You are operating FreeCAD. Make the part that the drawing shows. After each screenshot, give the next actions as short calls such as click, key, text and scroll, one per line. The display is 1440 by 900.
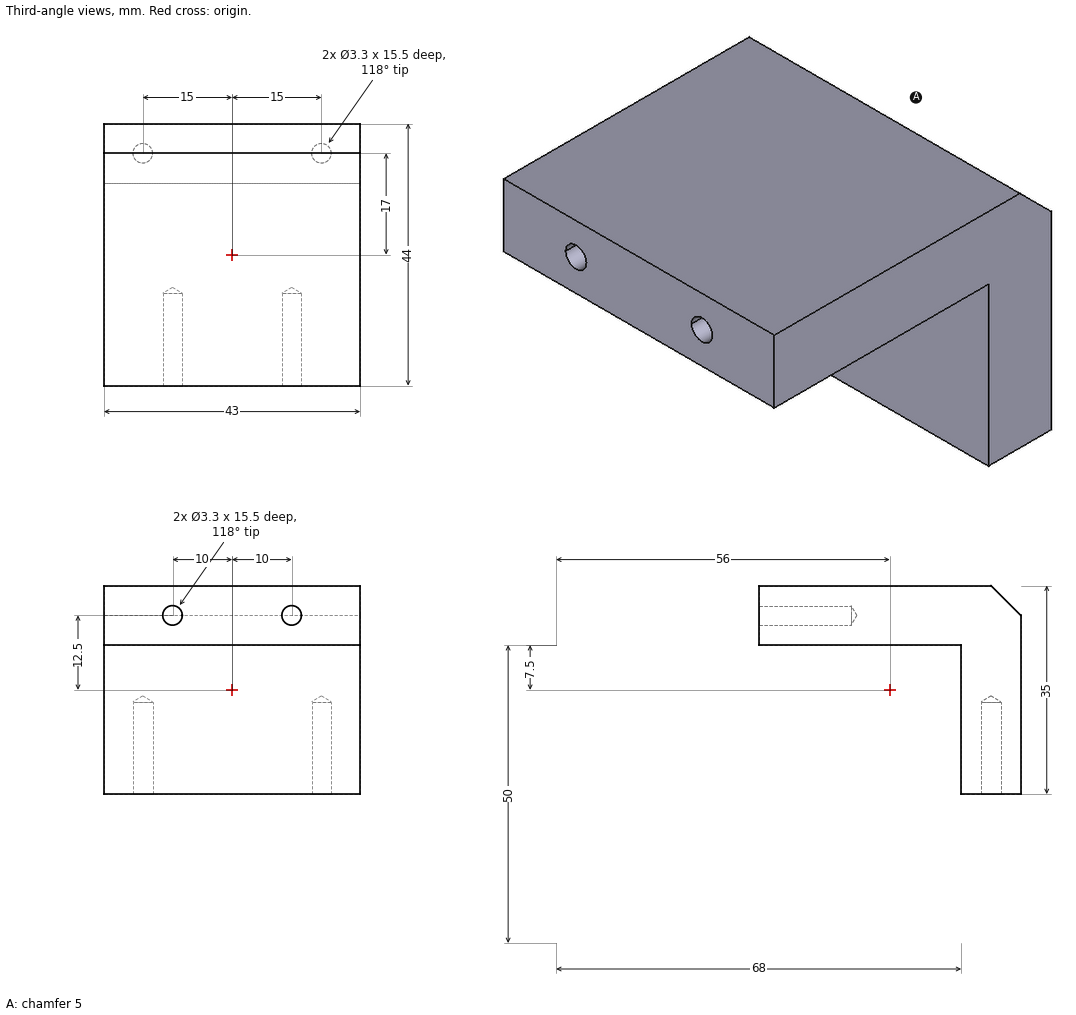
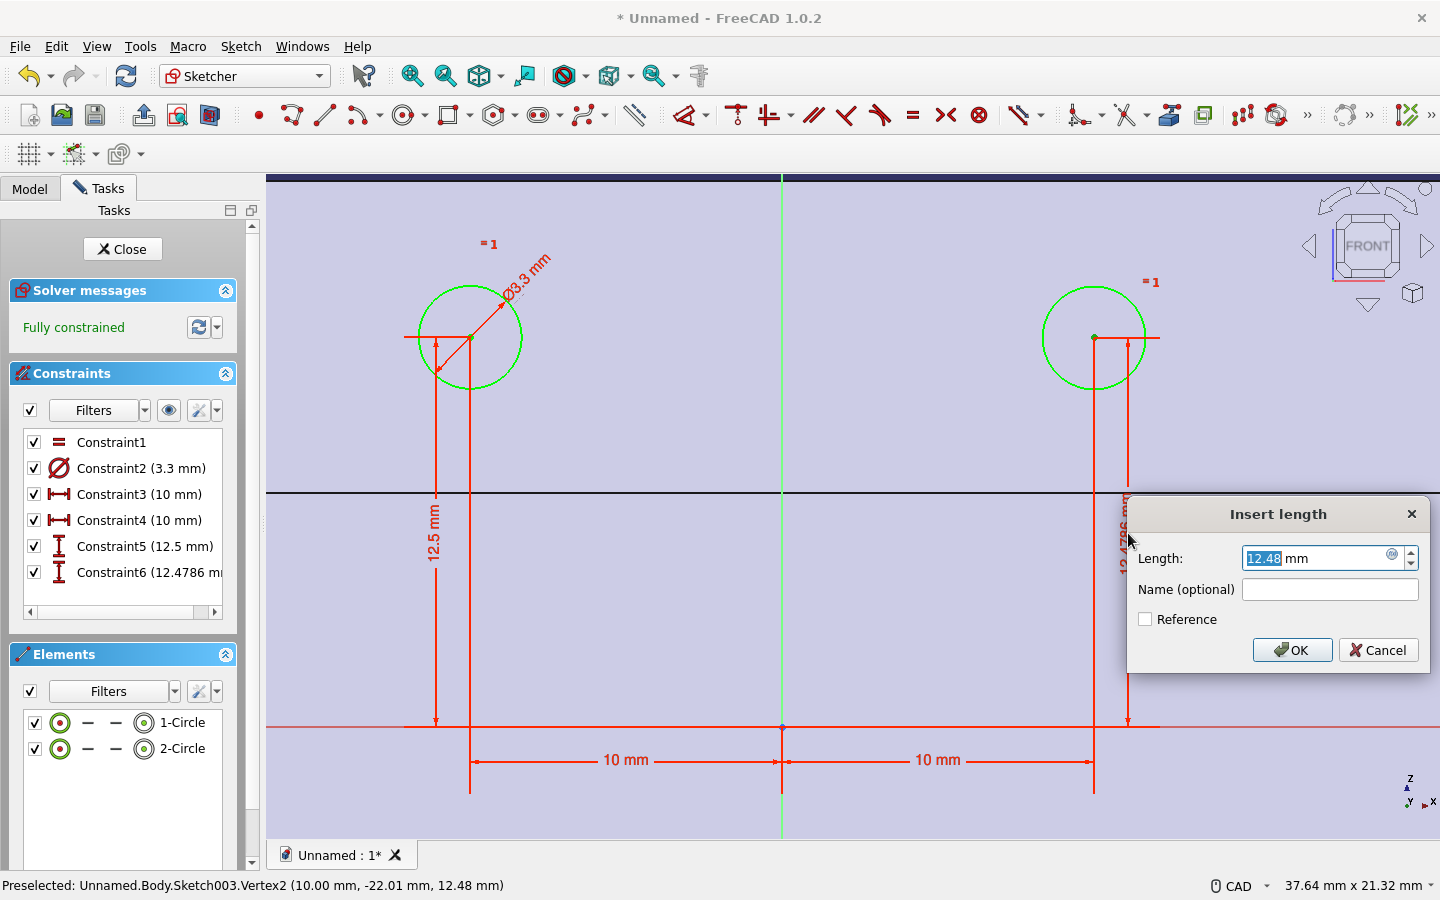
text(12.5)
key(Return)
key(Escape)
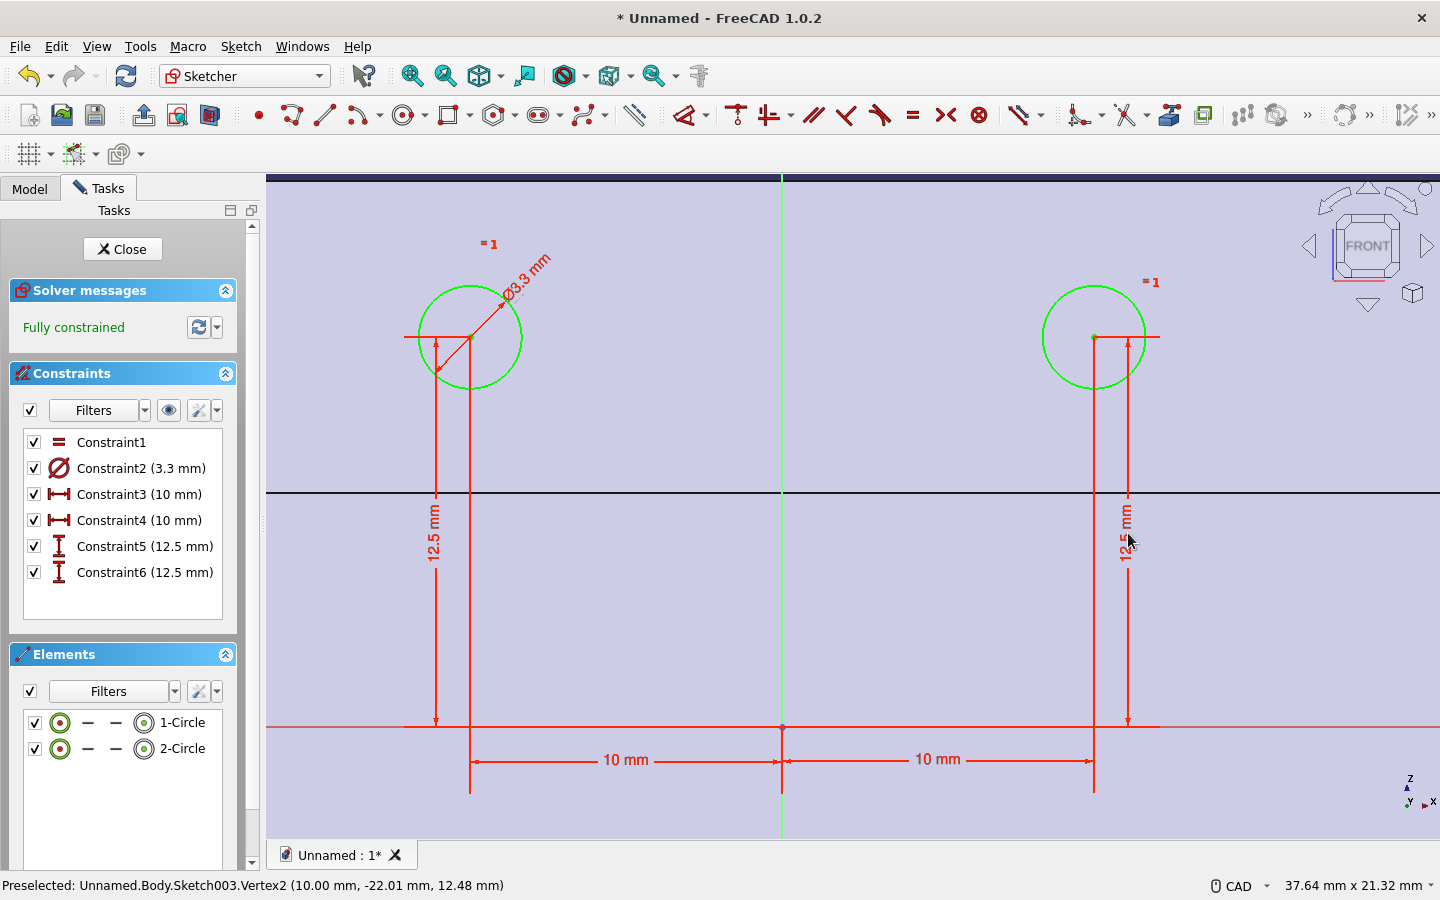
click(123, 249)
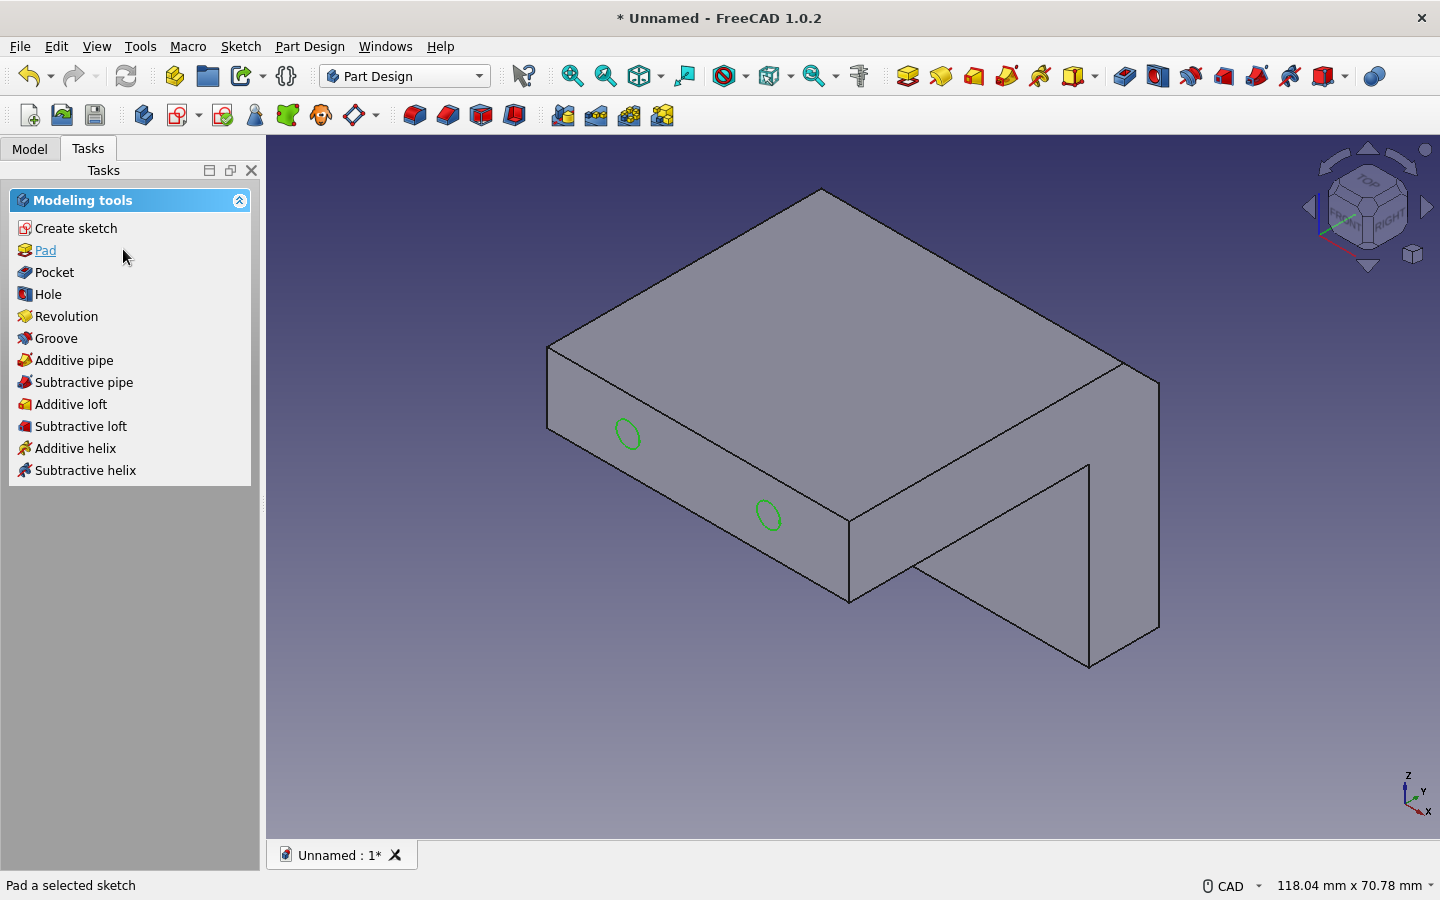
click(1158, 76)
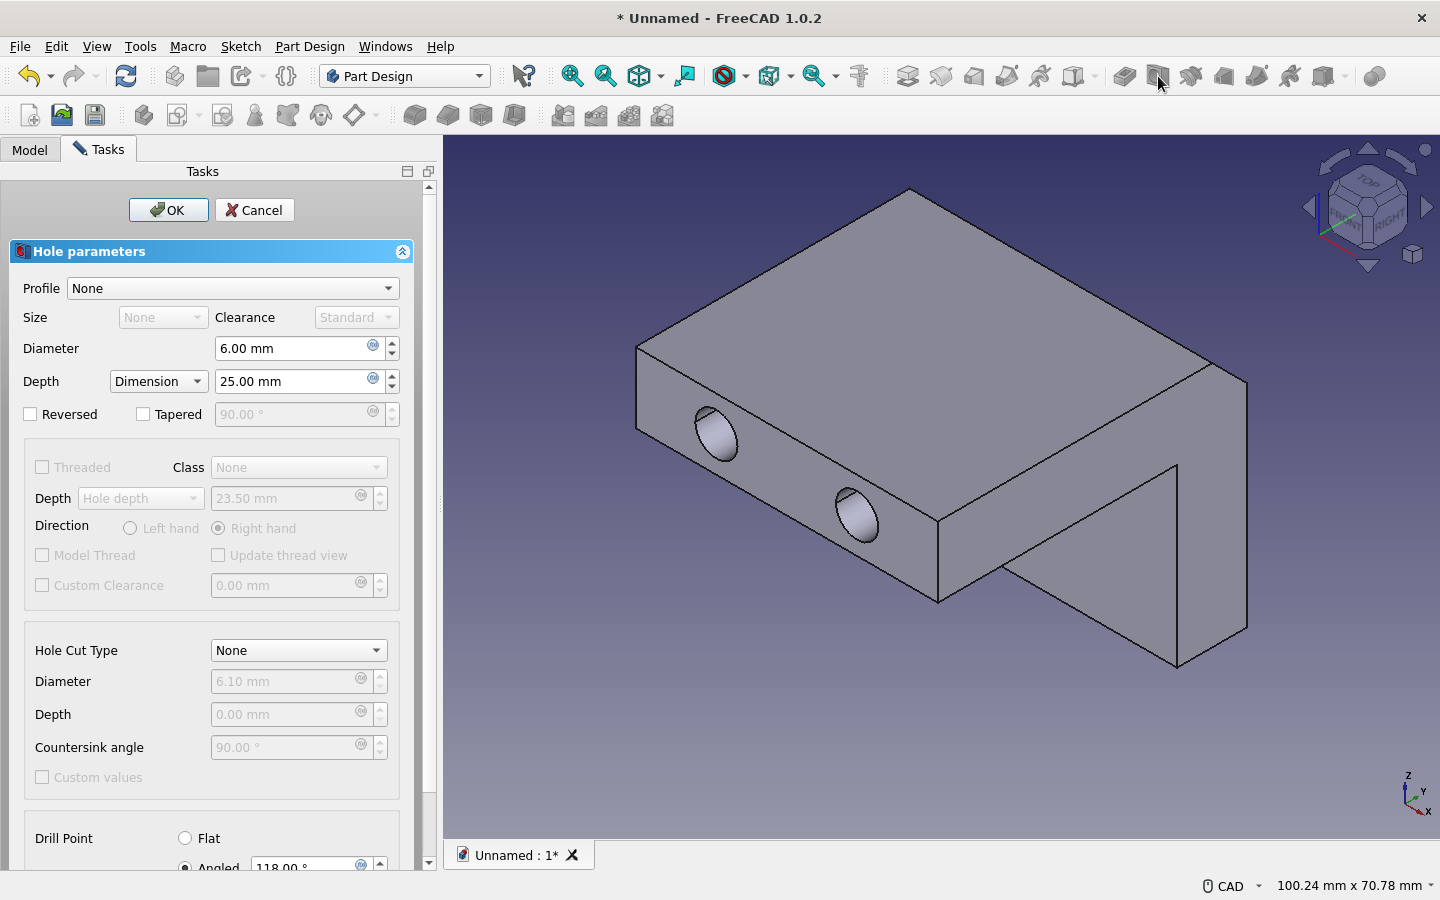
triple_click(300, 348)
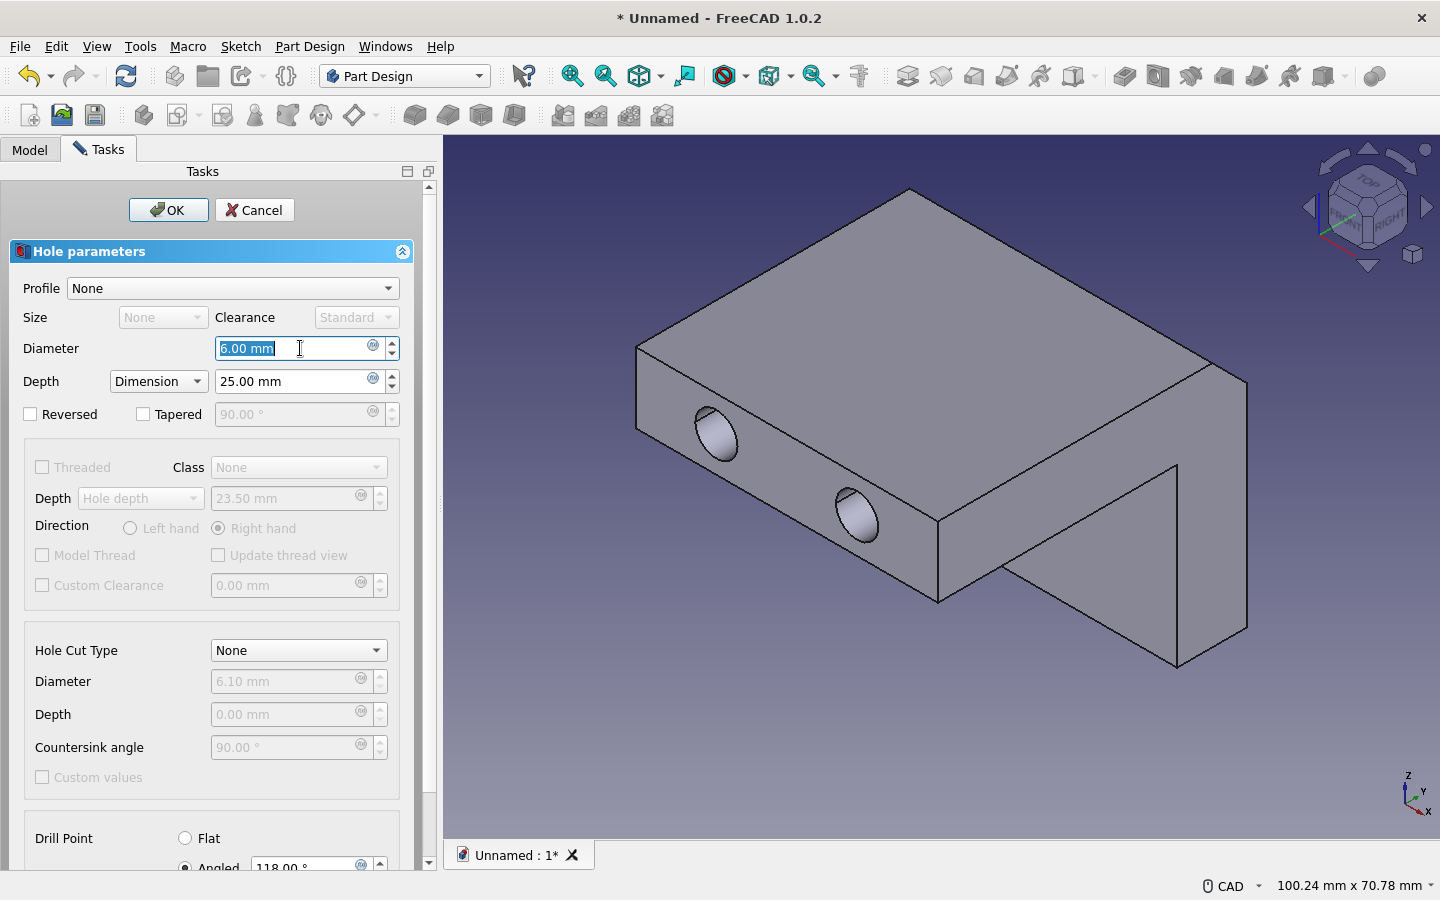
text(3.3)
key(Tab)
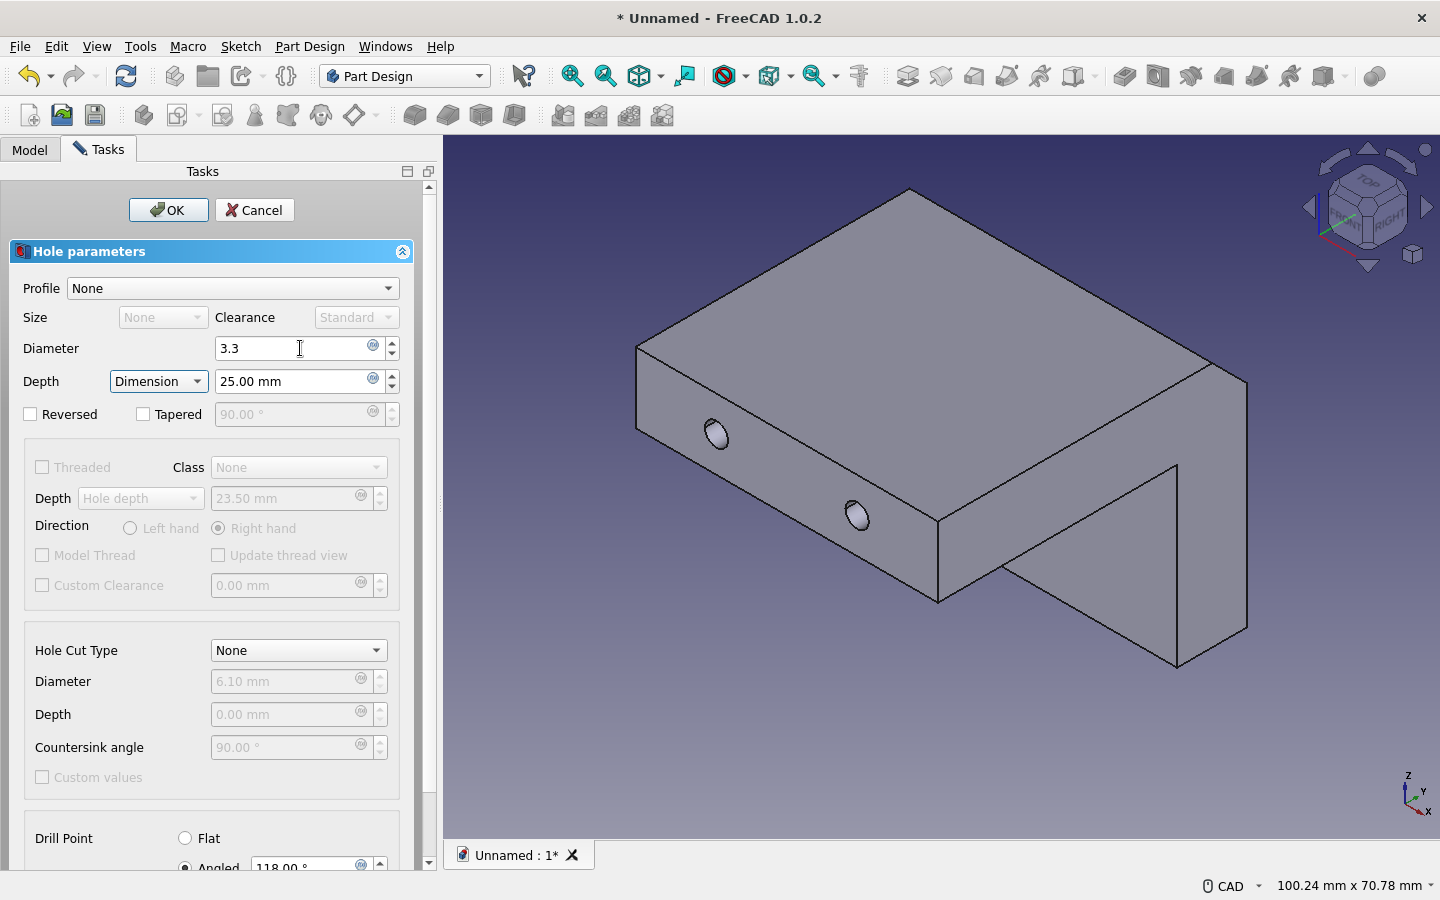
triple_click(300, 382)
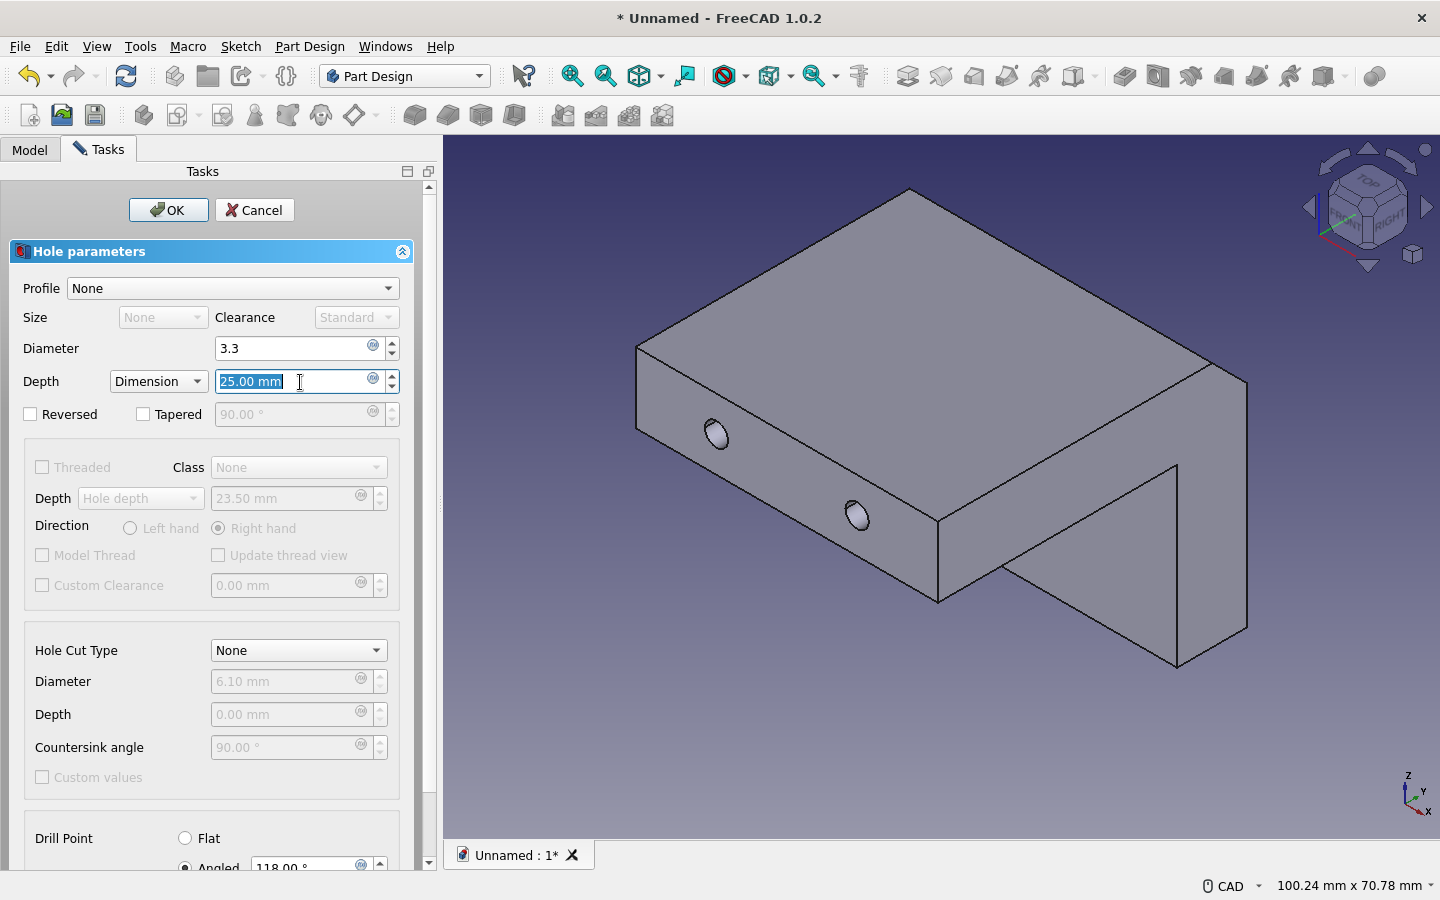
text(15.5)
key(Tab)